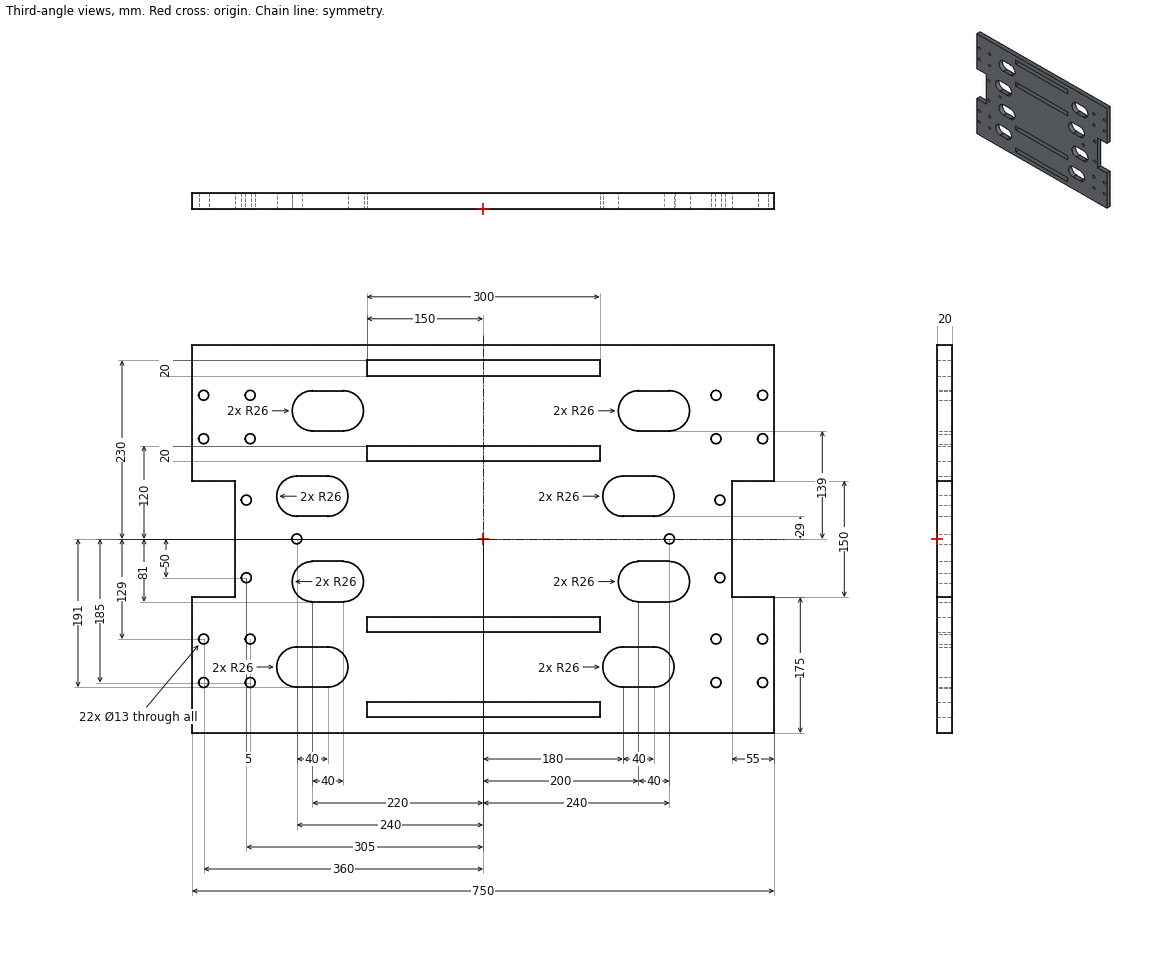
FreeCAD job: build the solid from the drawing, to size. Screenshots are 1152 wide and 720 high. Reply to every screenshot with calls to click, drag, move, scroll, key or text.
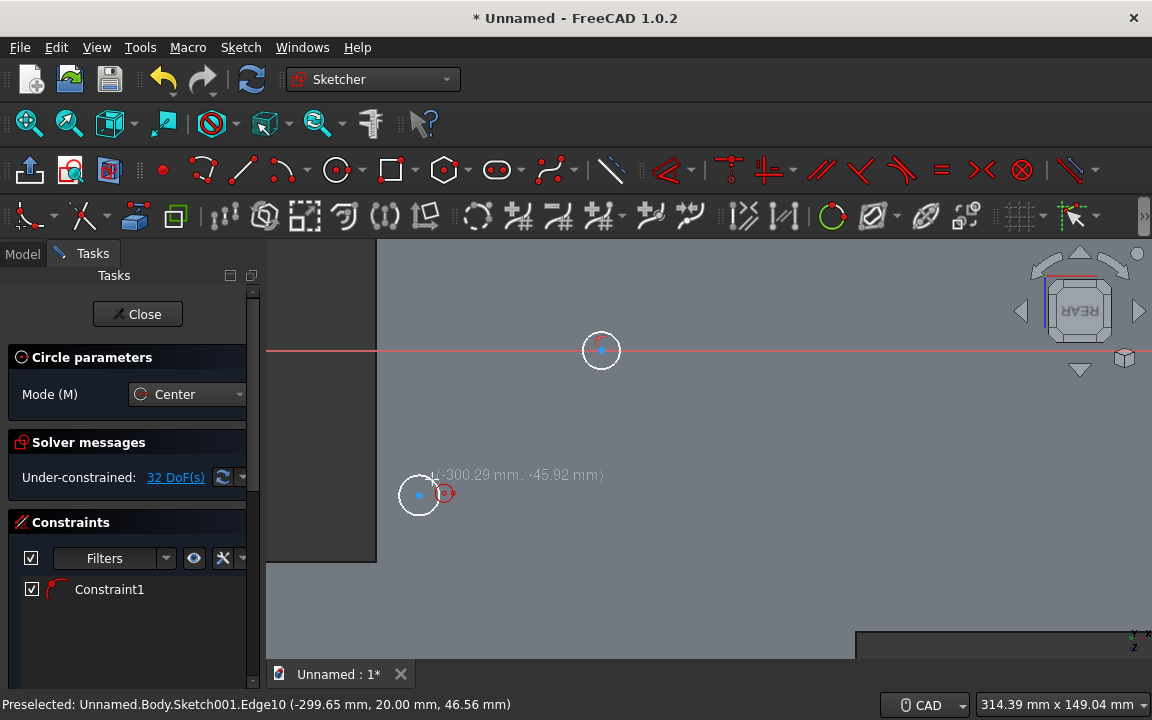
scroll(432, 481, down, 7)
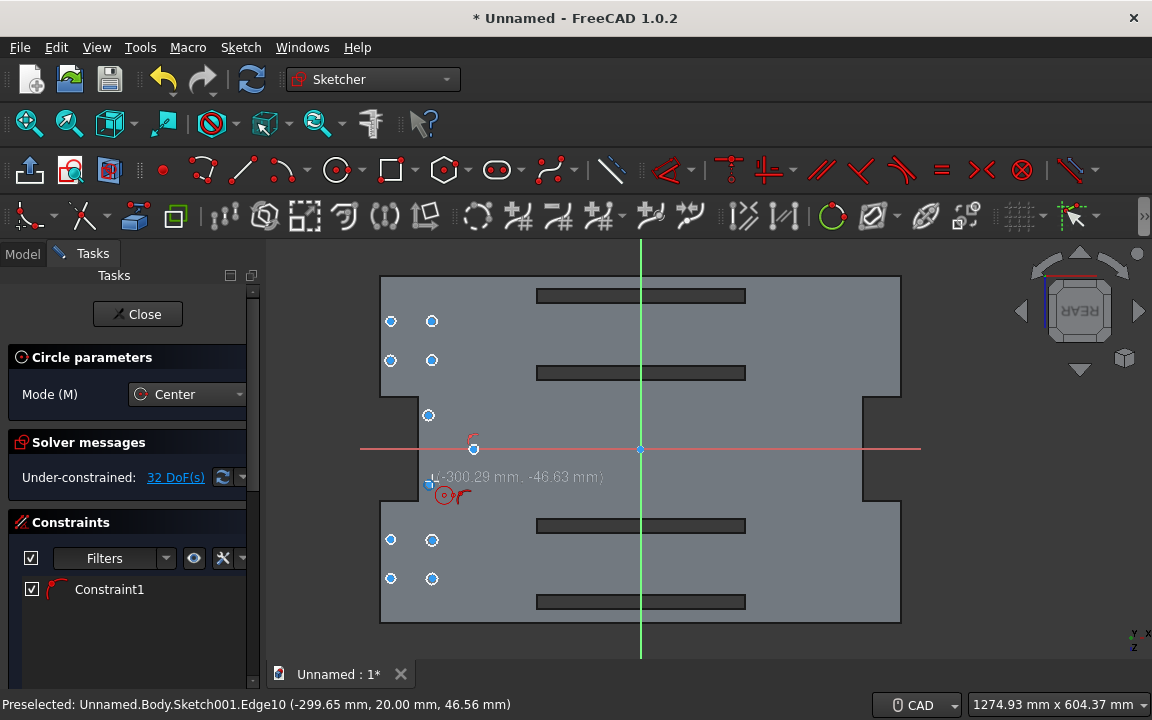
scroll(891, 539, up, 9)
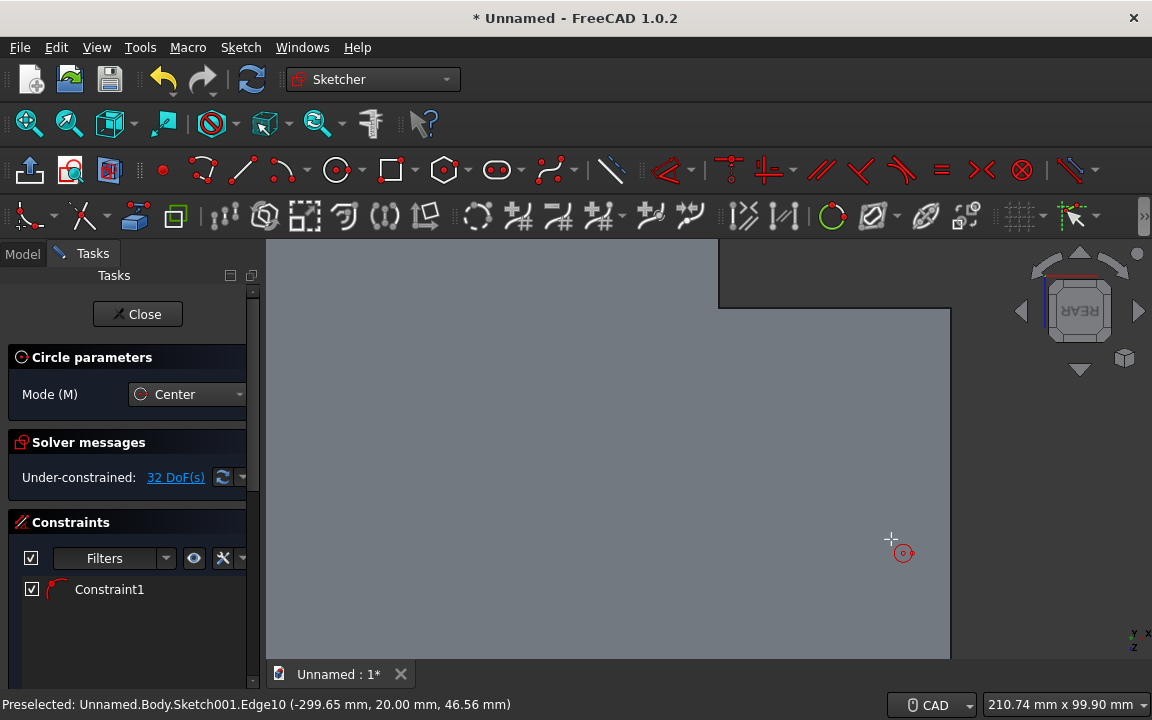
scroll(891, 539, down, 9)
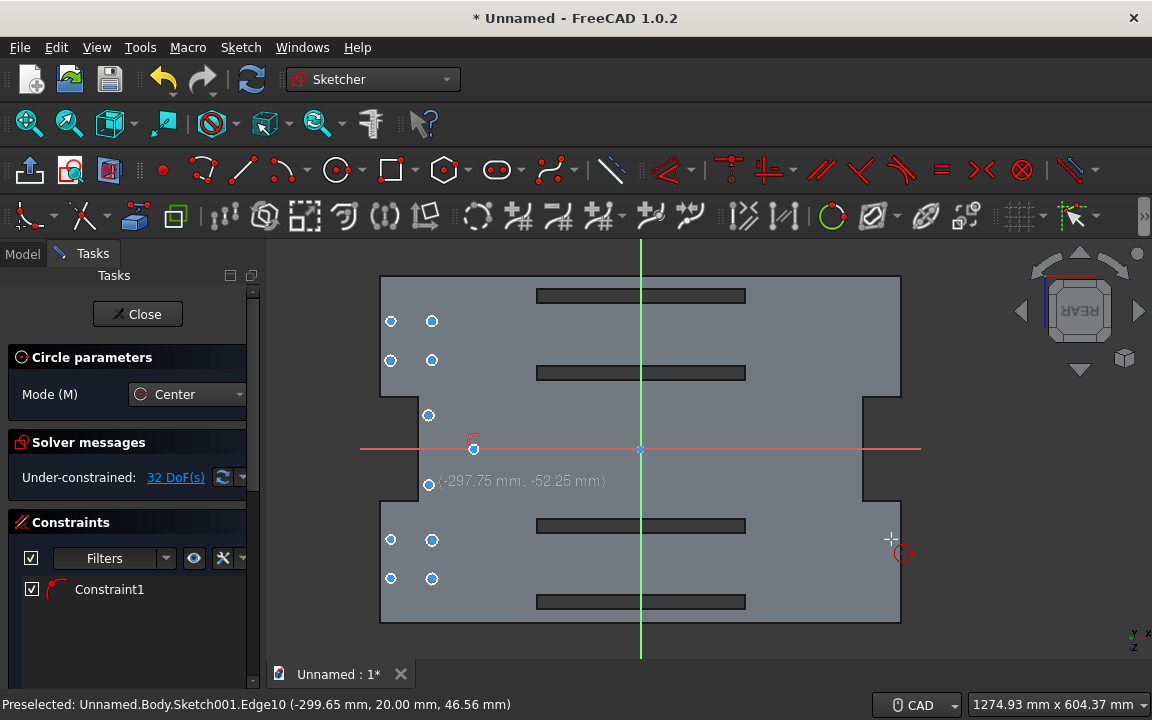
click(891, 539)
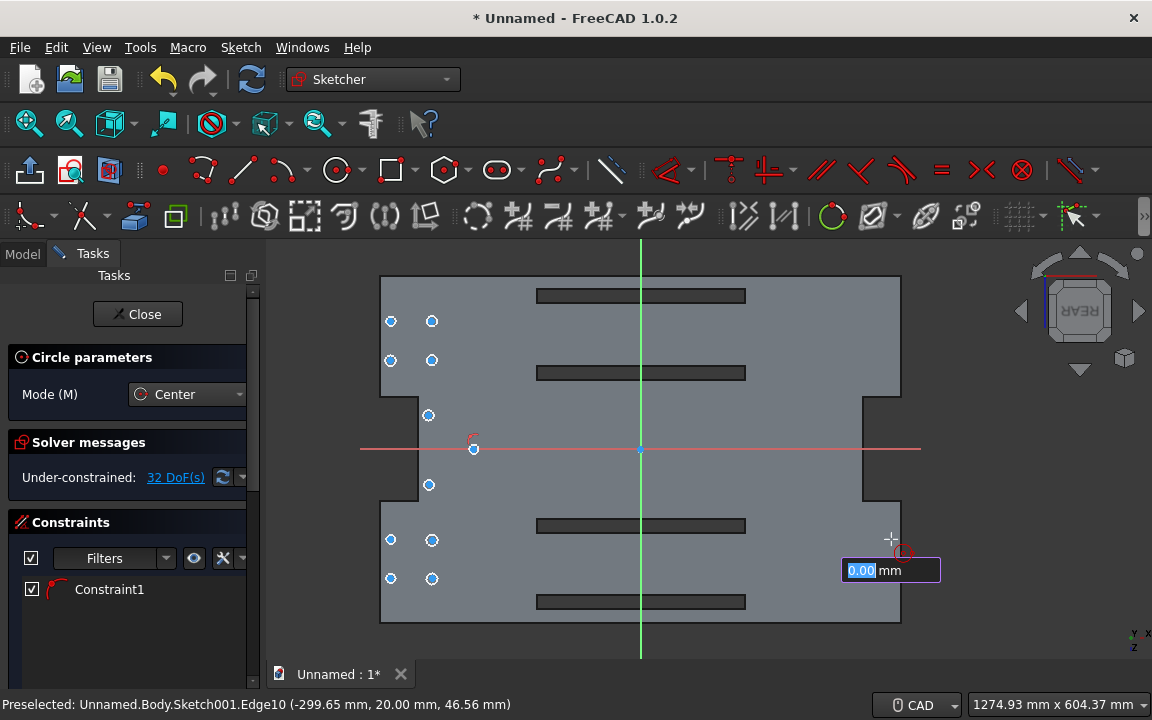
scroll(894, 536, up, 7)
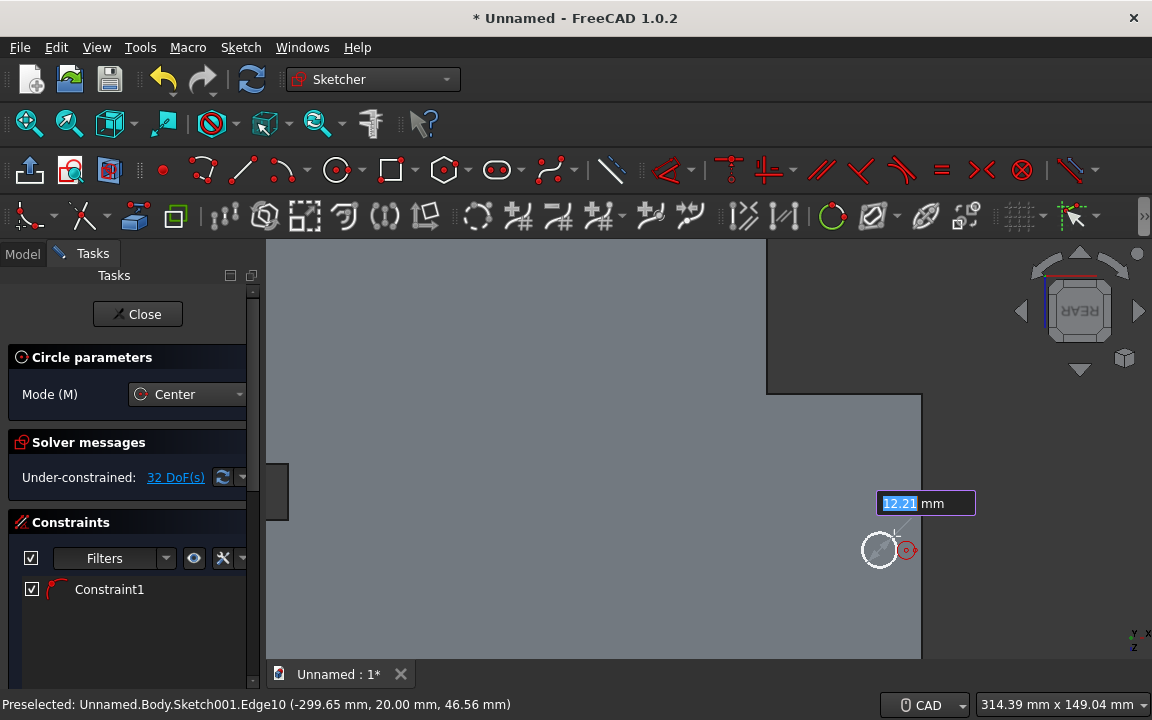
click(893, 533)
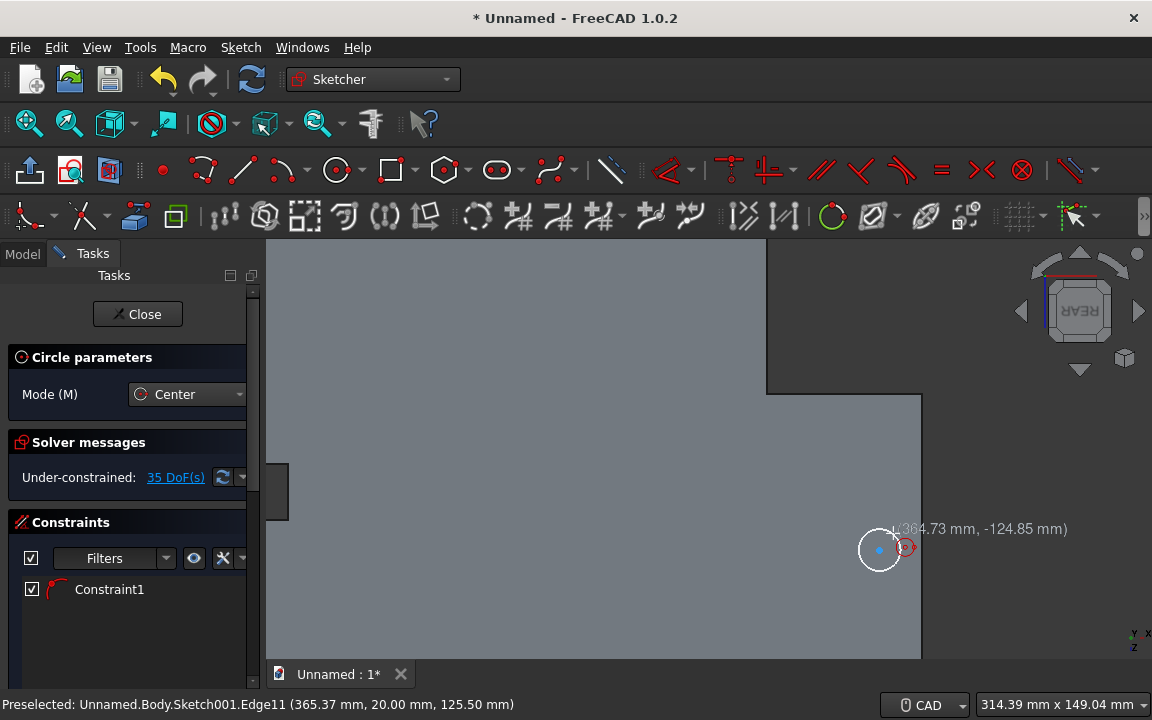
scroll(711, 546, up, 2)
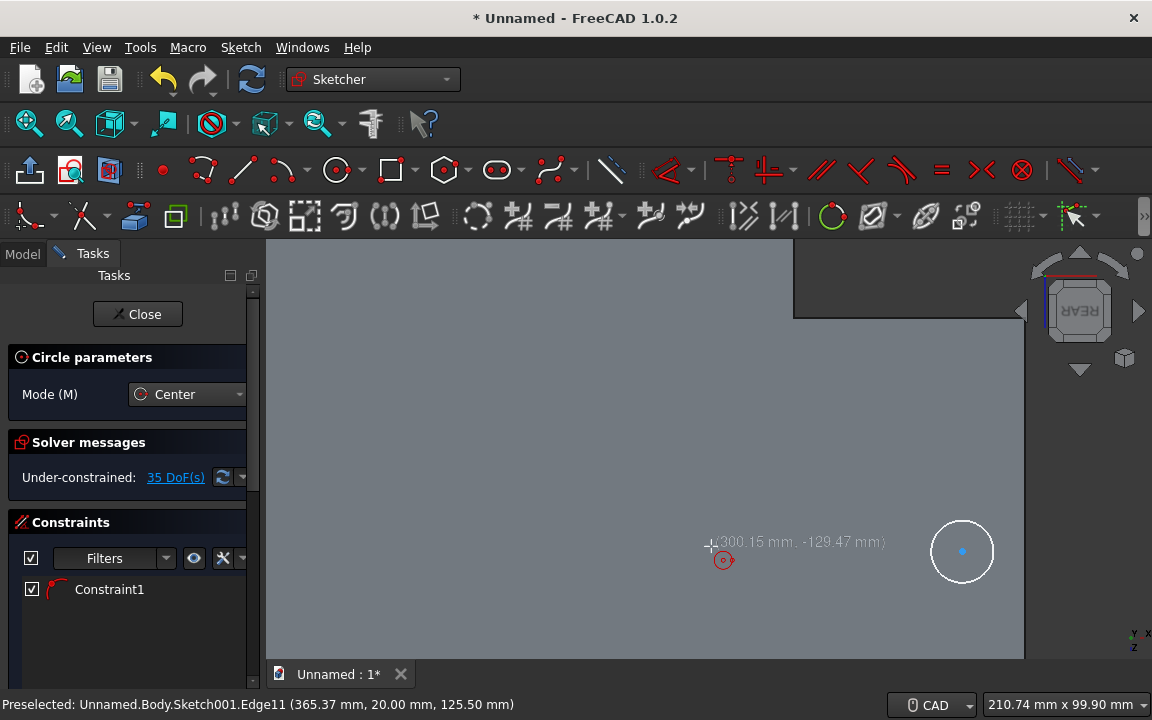
scroll(876, 537, down, 9)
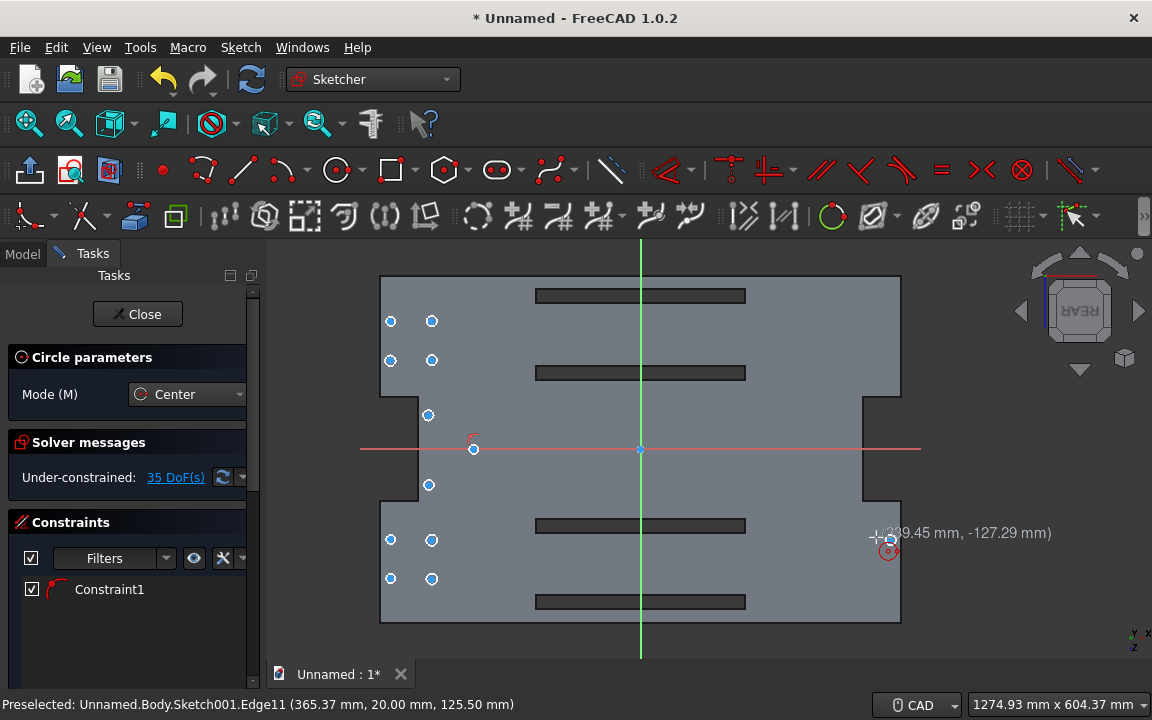
click(849, 539)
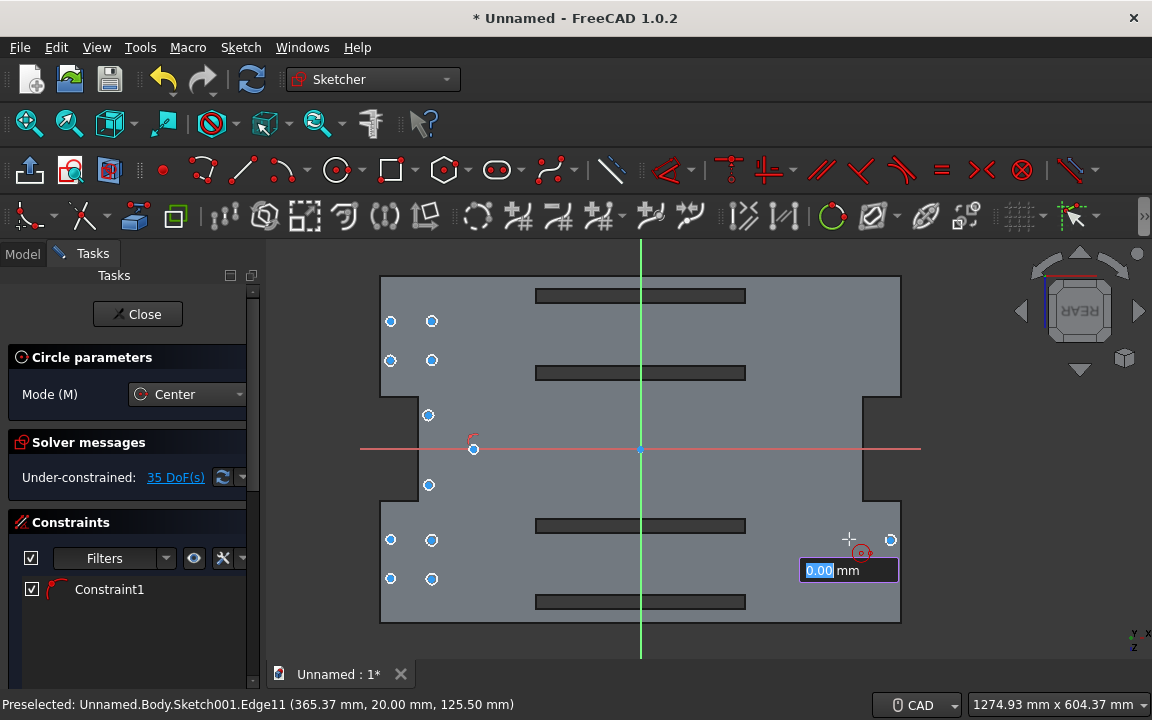
scroll(852, 536, up, 7)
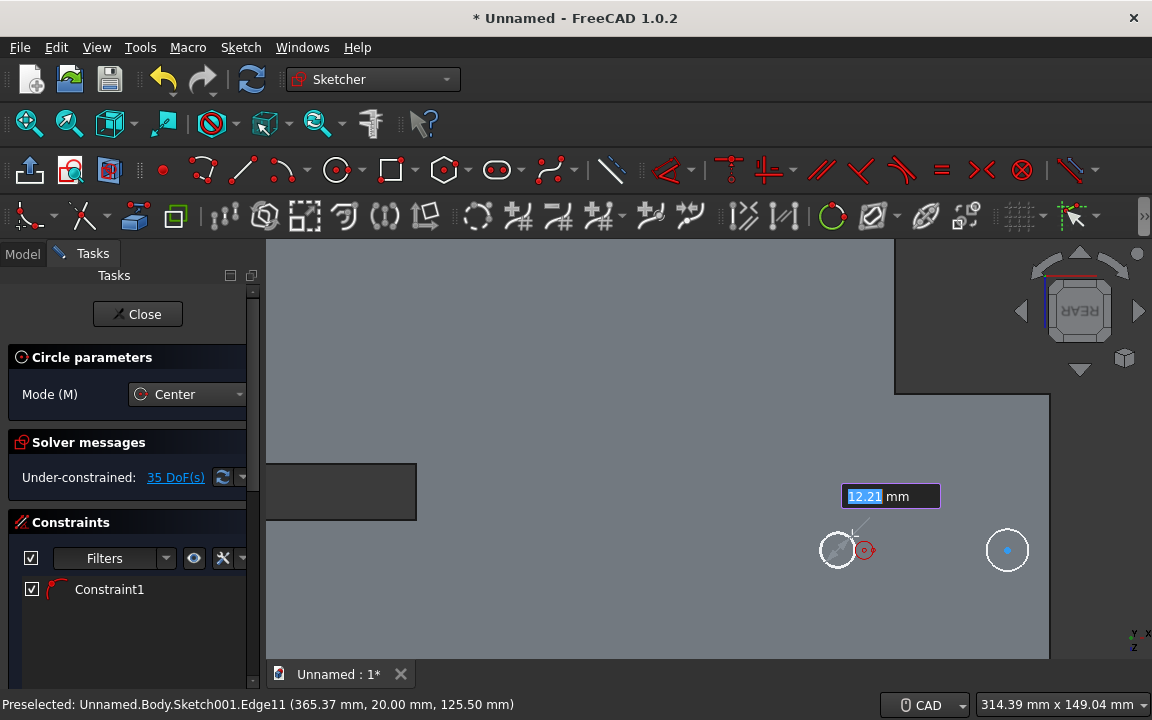
click(851, 533)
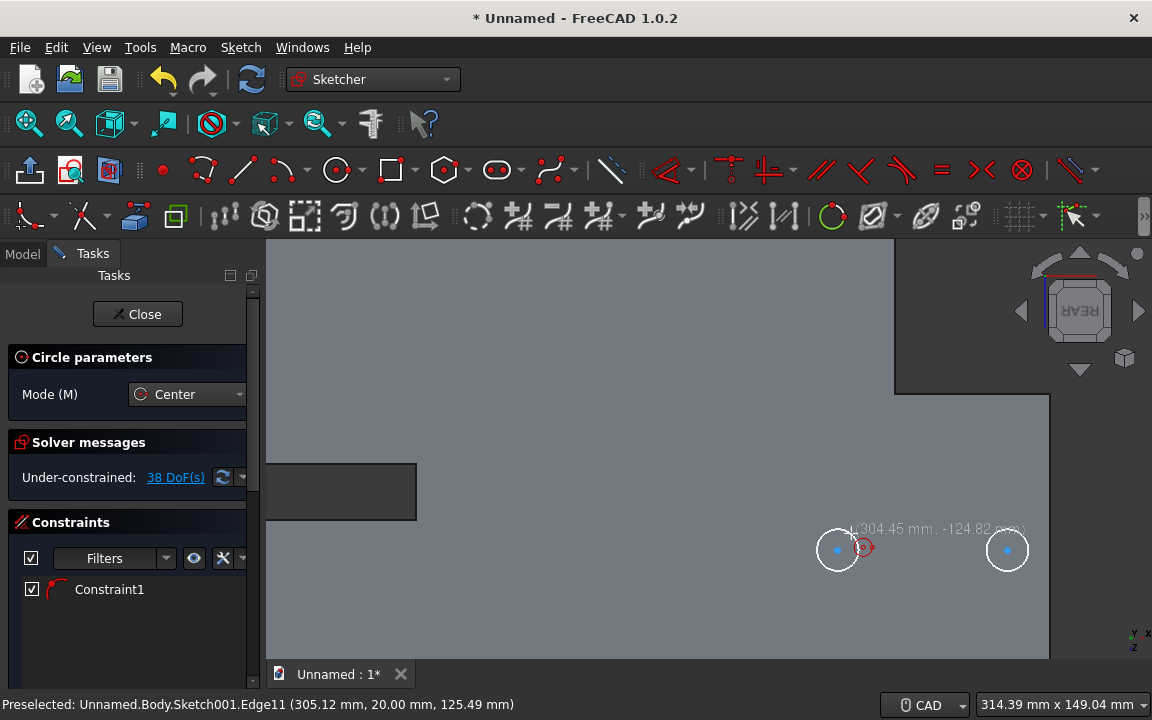
scroll(852, 536, down, 7)